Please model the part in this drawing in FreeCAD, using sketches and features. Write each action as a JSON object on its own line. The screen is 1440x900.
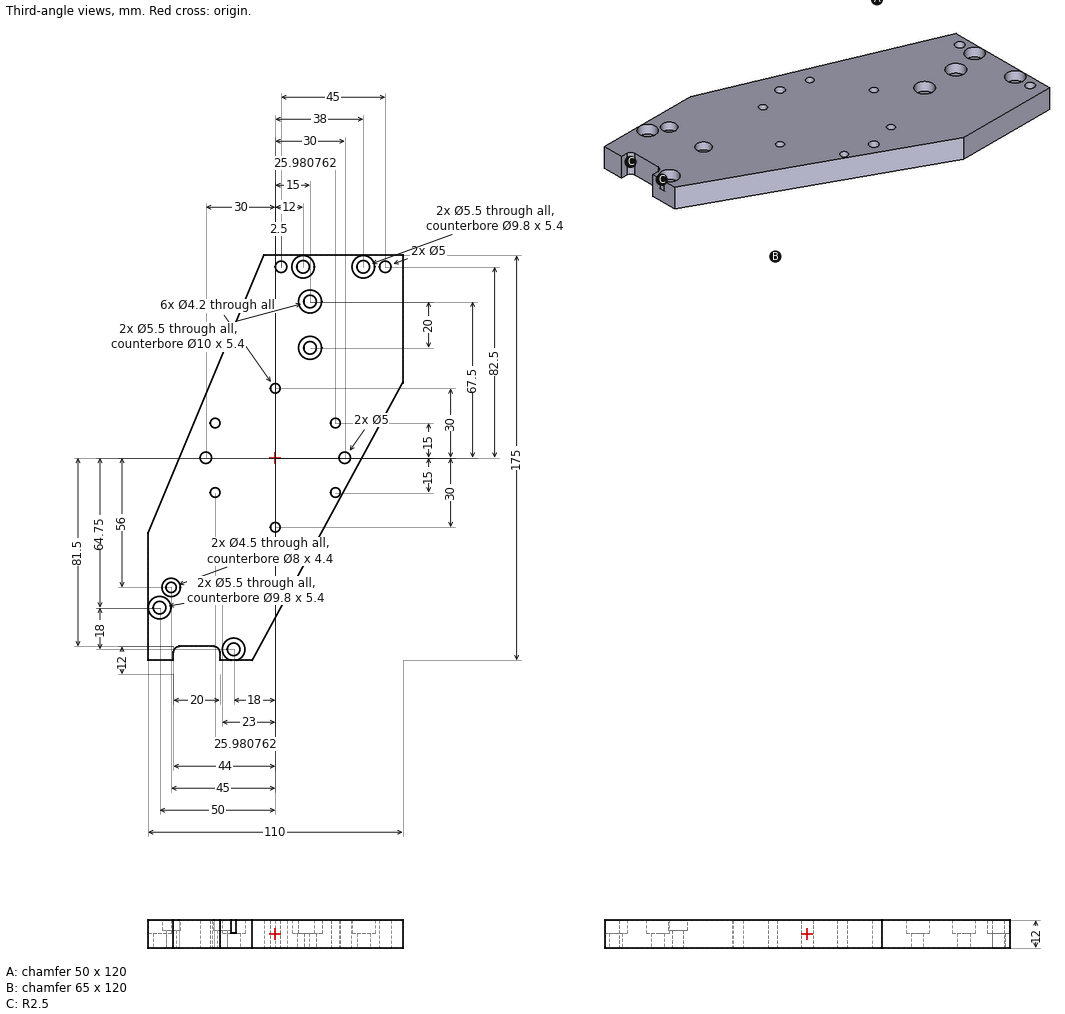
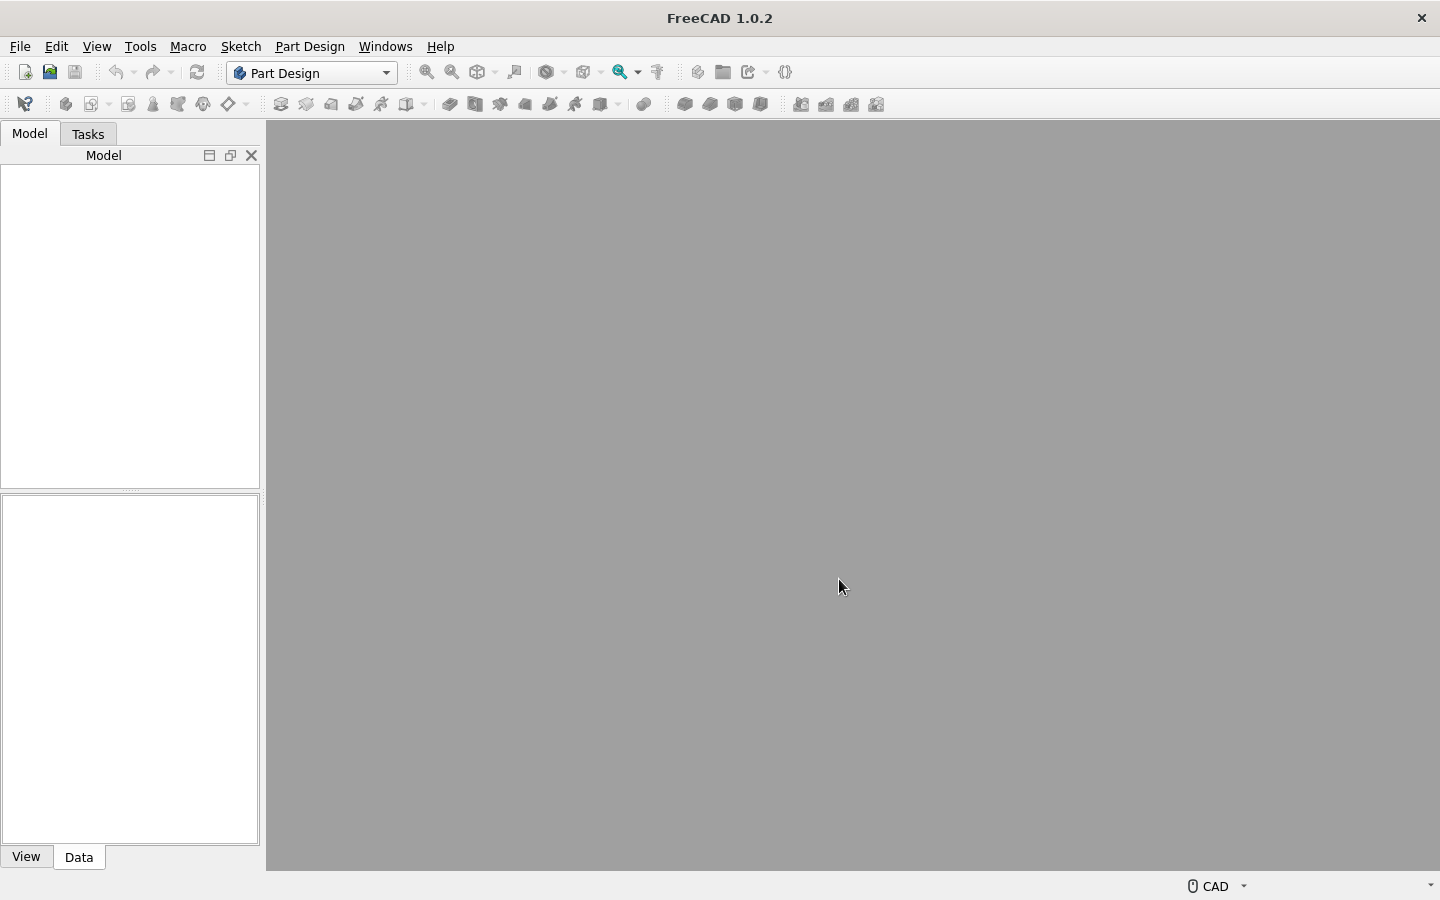
{"action": "key", "text": "ctrl+n"}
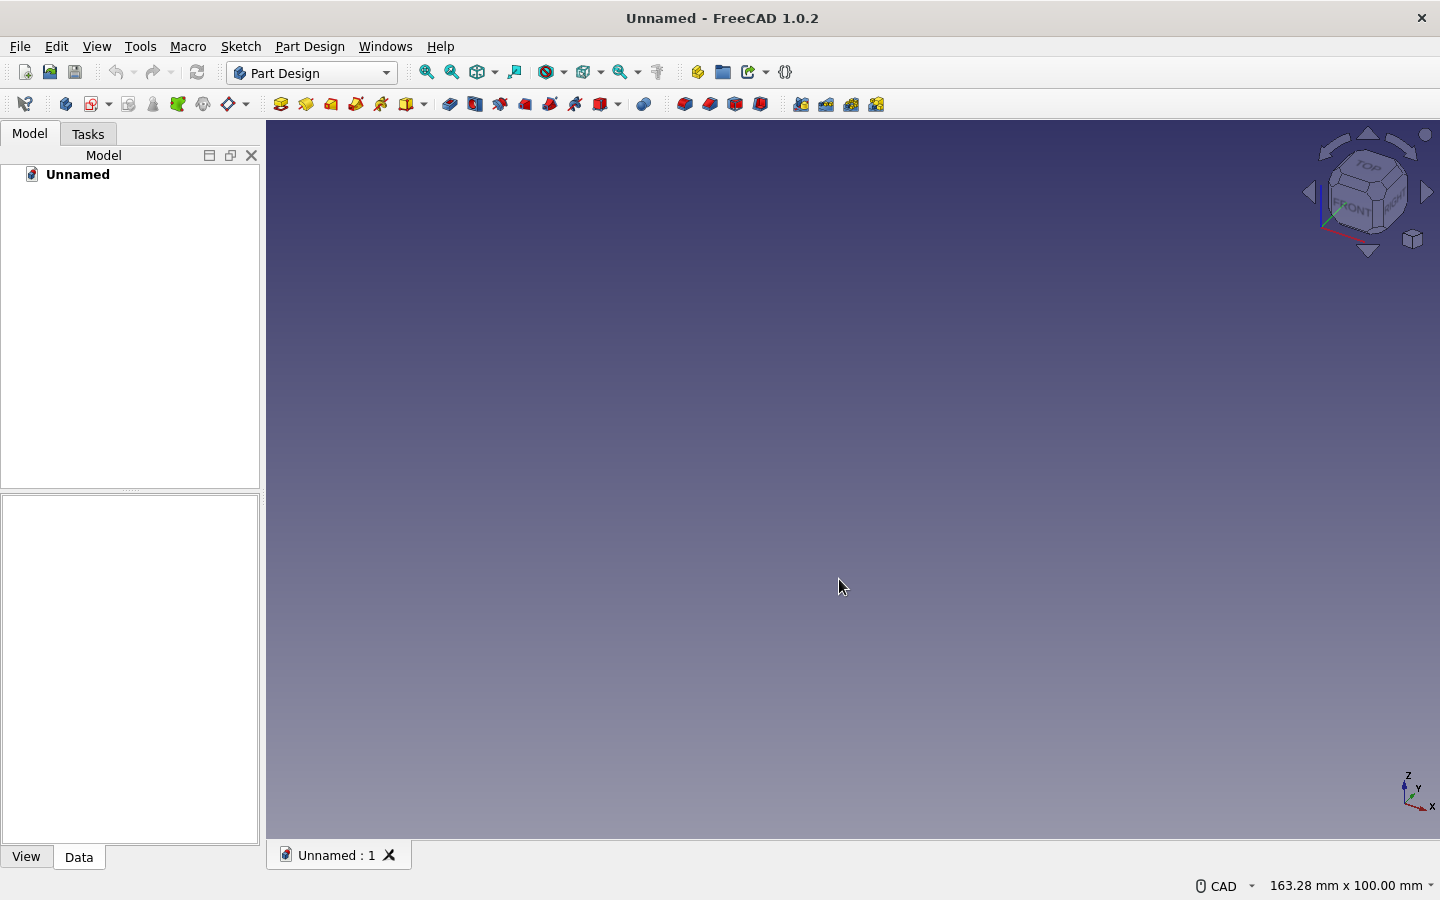
{"action": "left_click", "coordinate": [90, 104]}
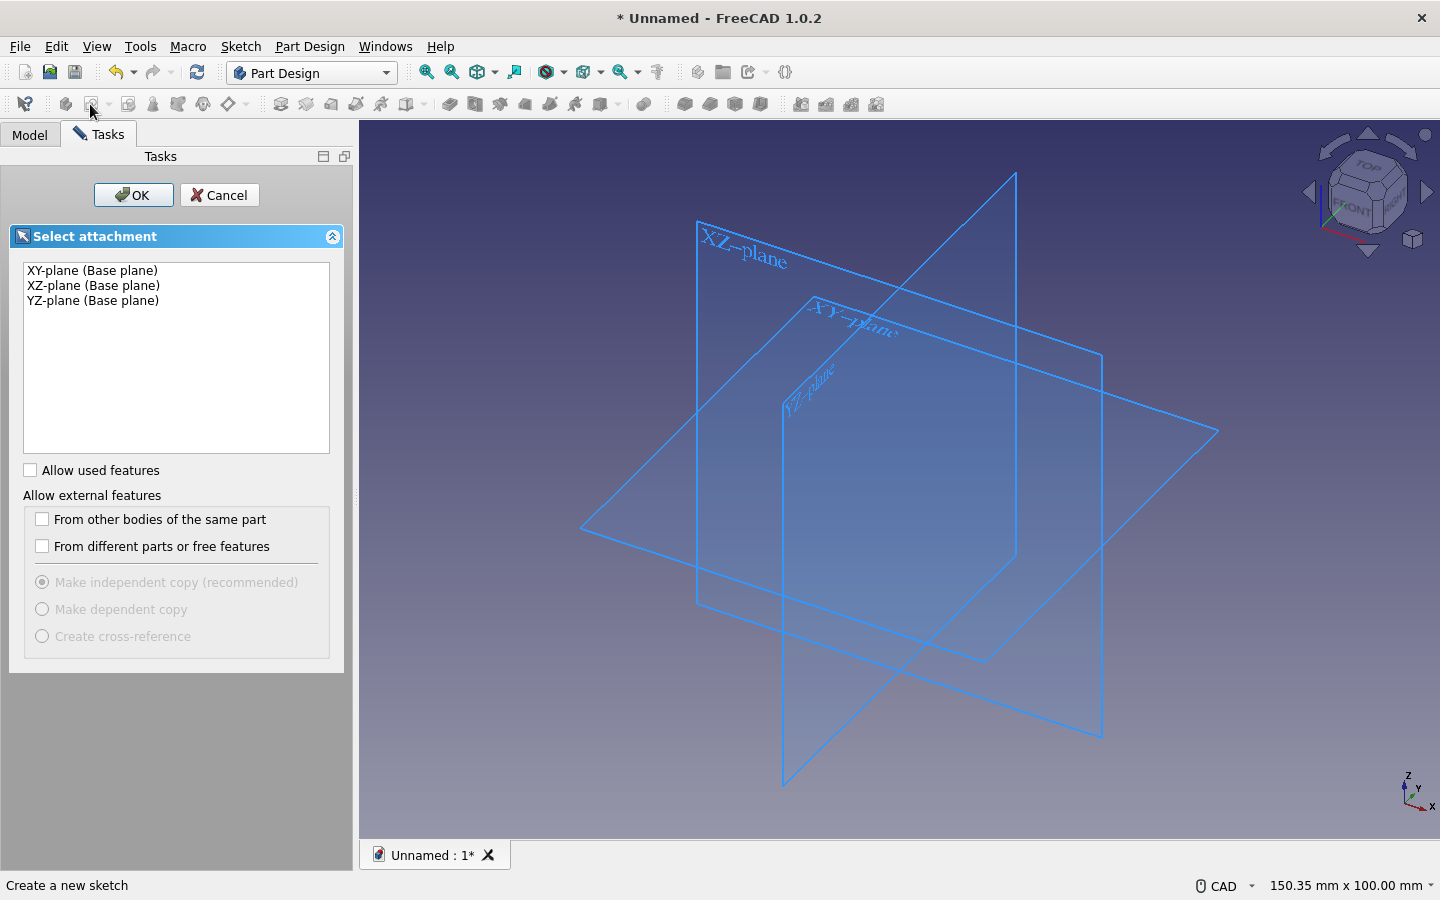
{"action": "left_click", "coordinate": [84, 270]}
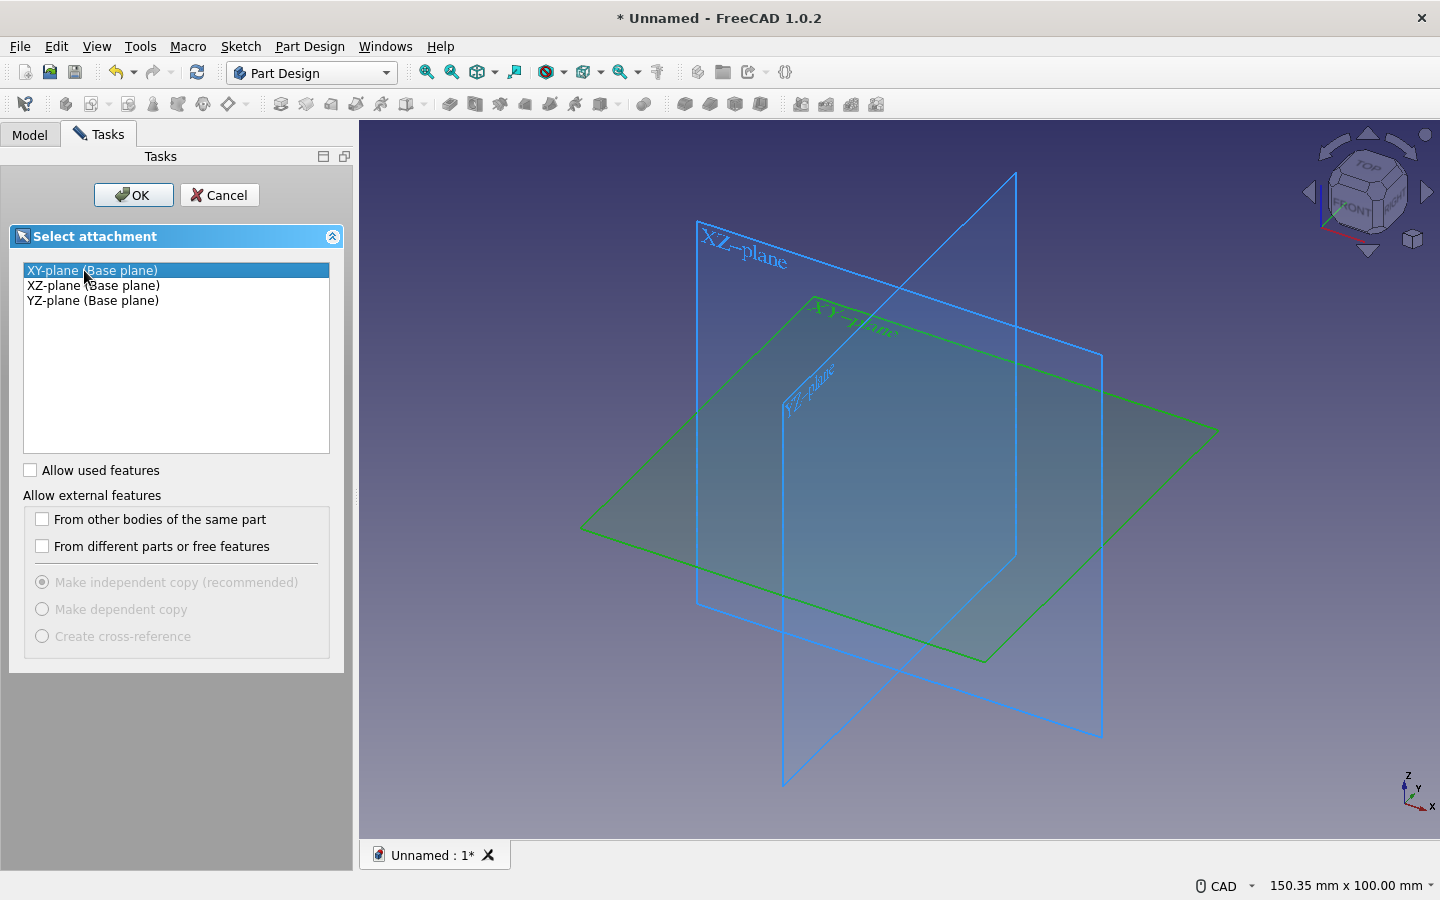
{"action": "left_click", "coordinate": [134, 195]}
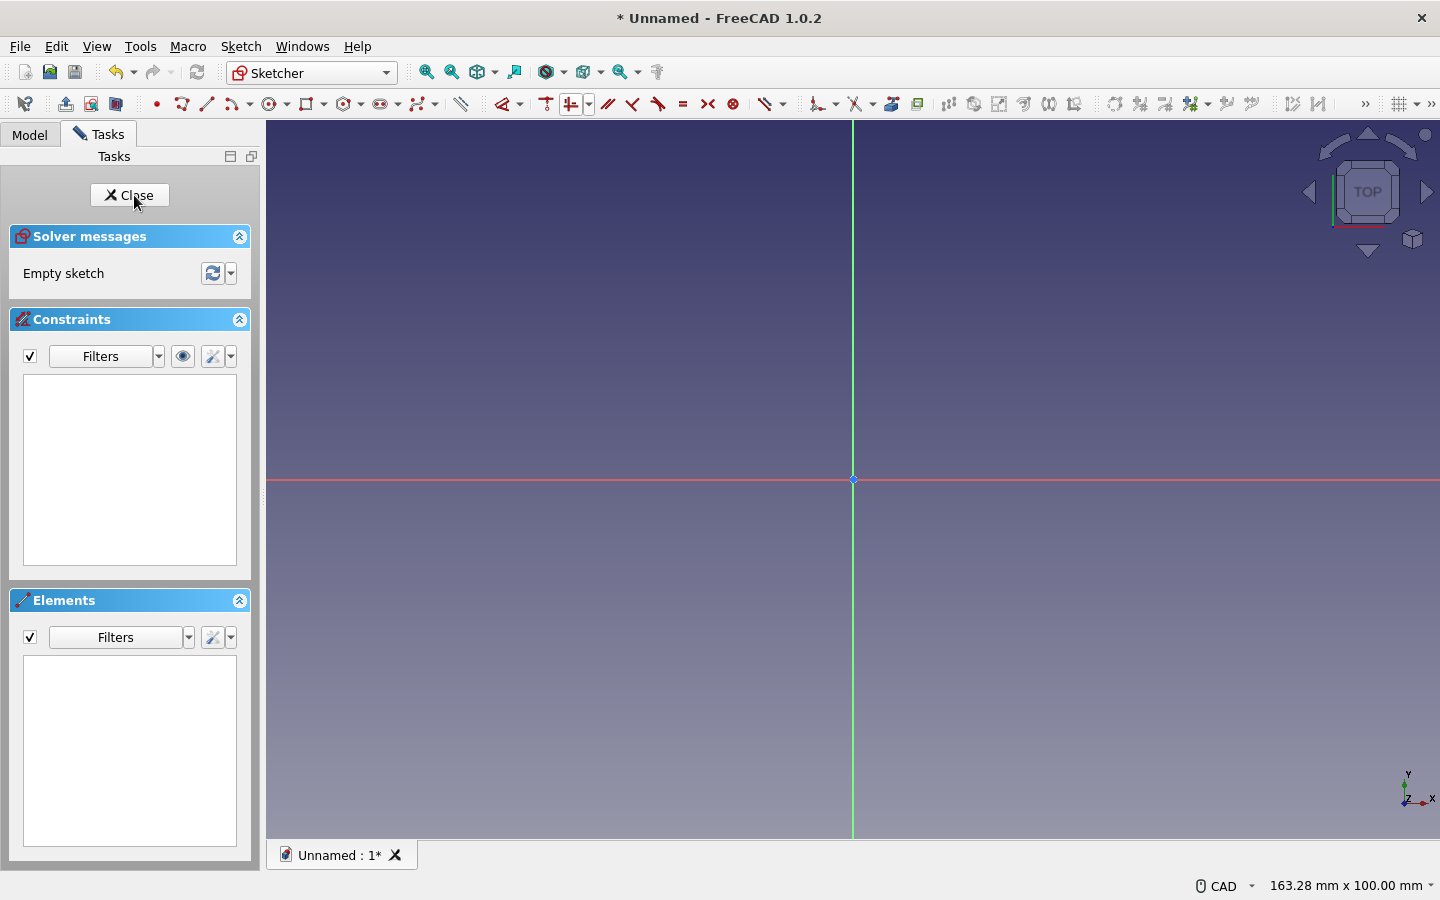
{"action": "scroll", "coordinate": [745, 480], "scroll_direction": "down", "scroll_amount": 5}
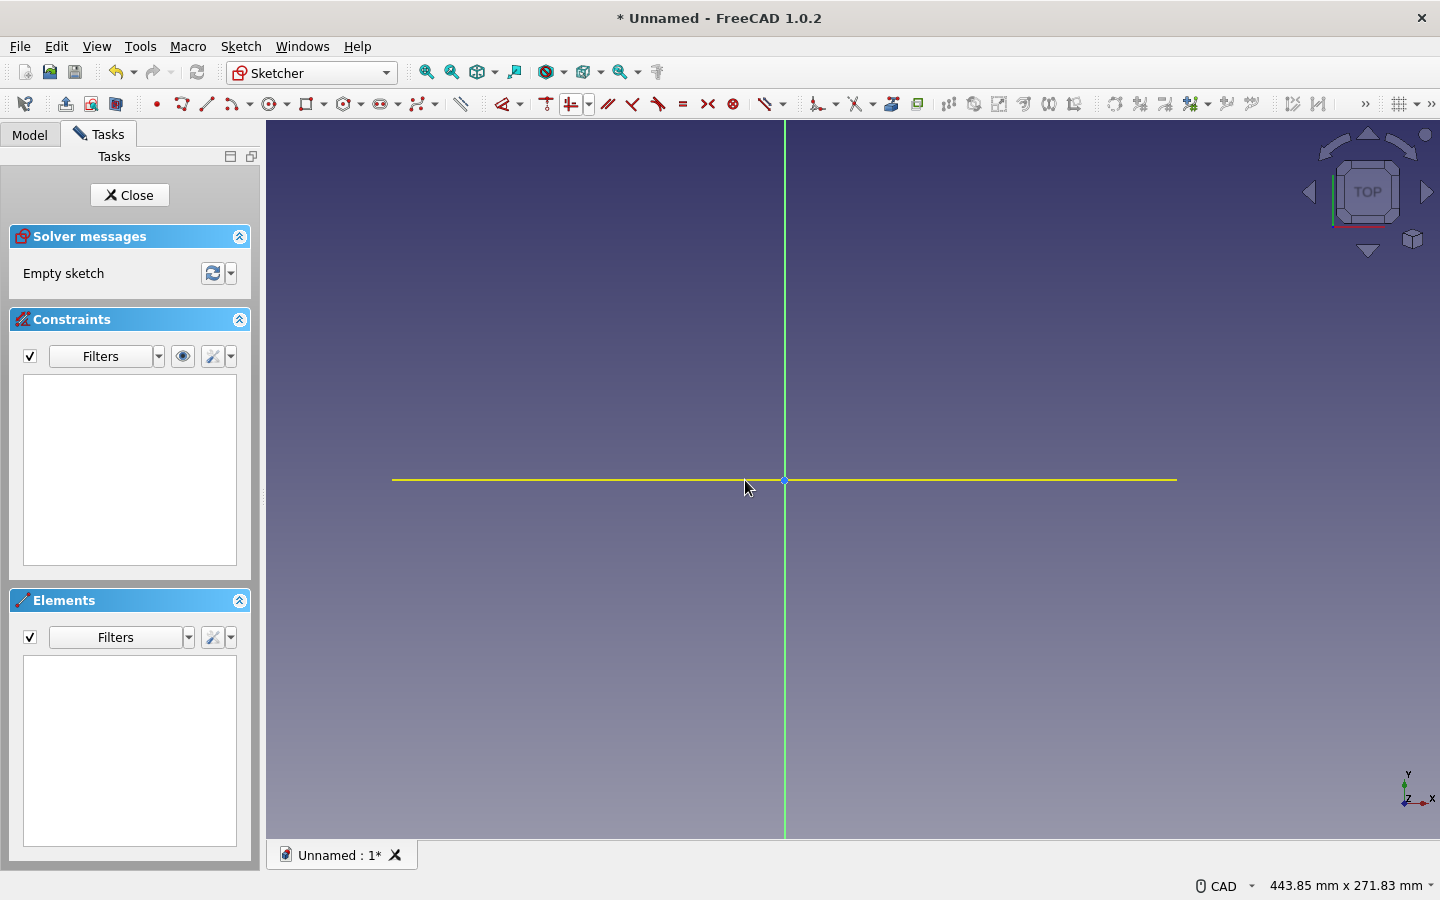
{"action": "left_click", "coordinate": [324, 104]}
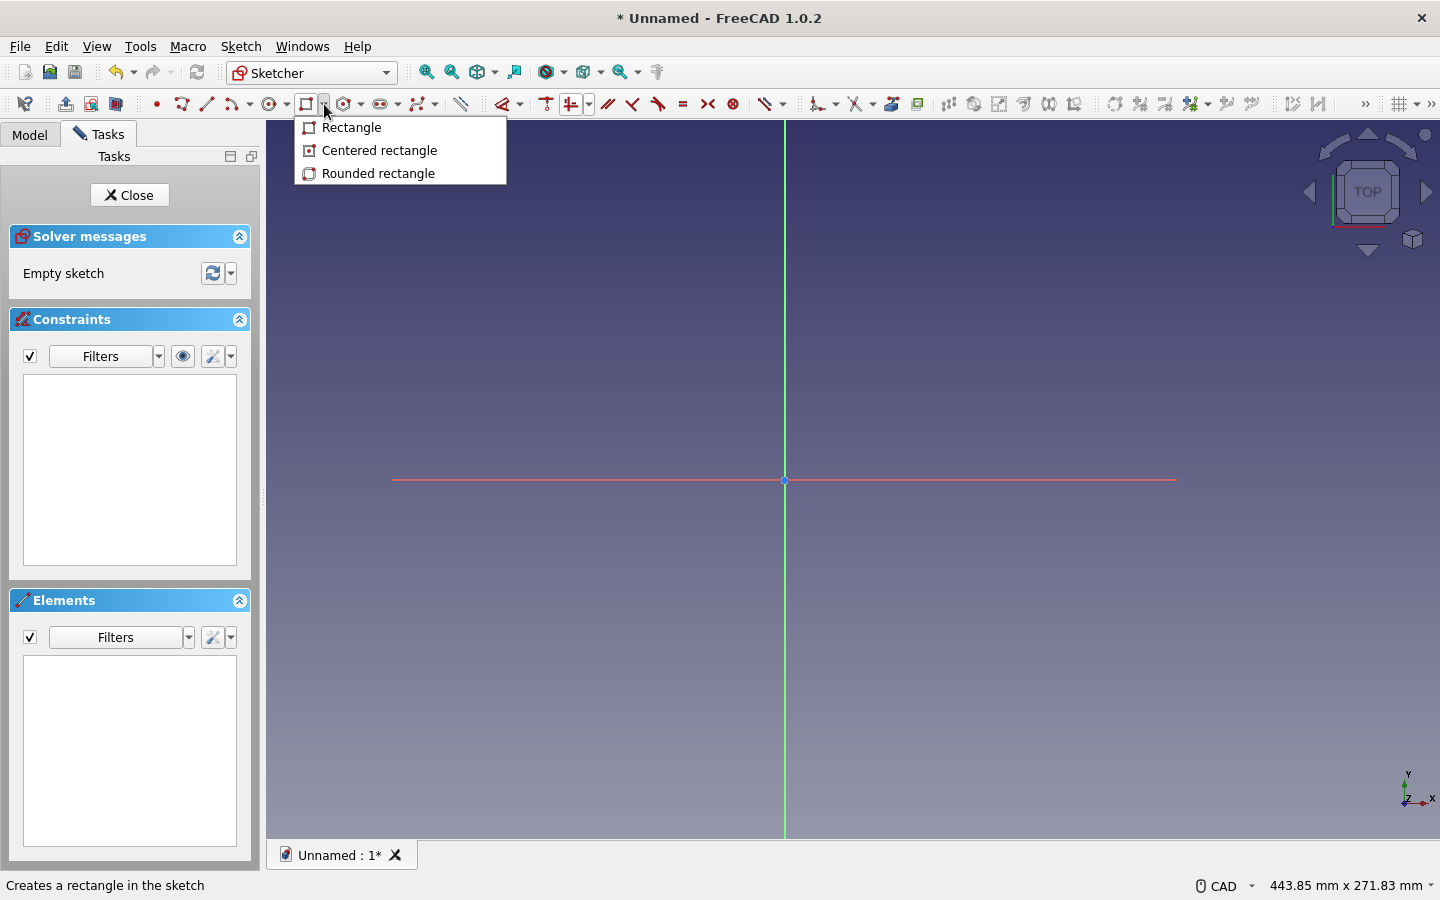
{"action": "left_click", "coordinate": [400, 150]}